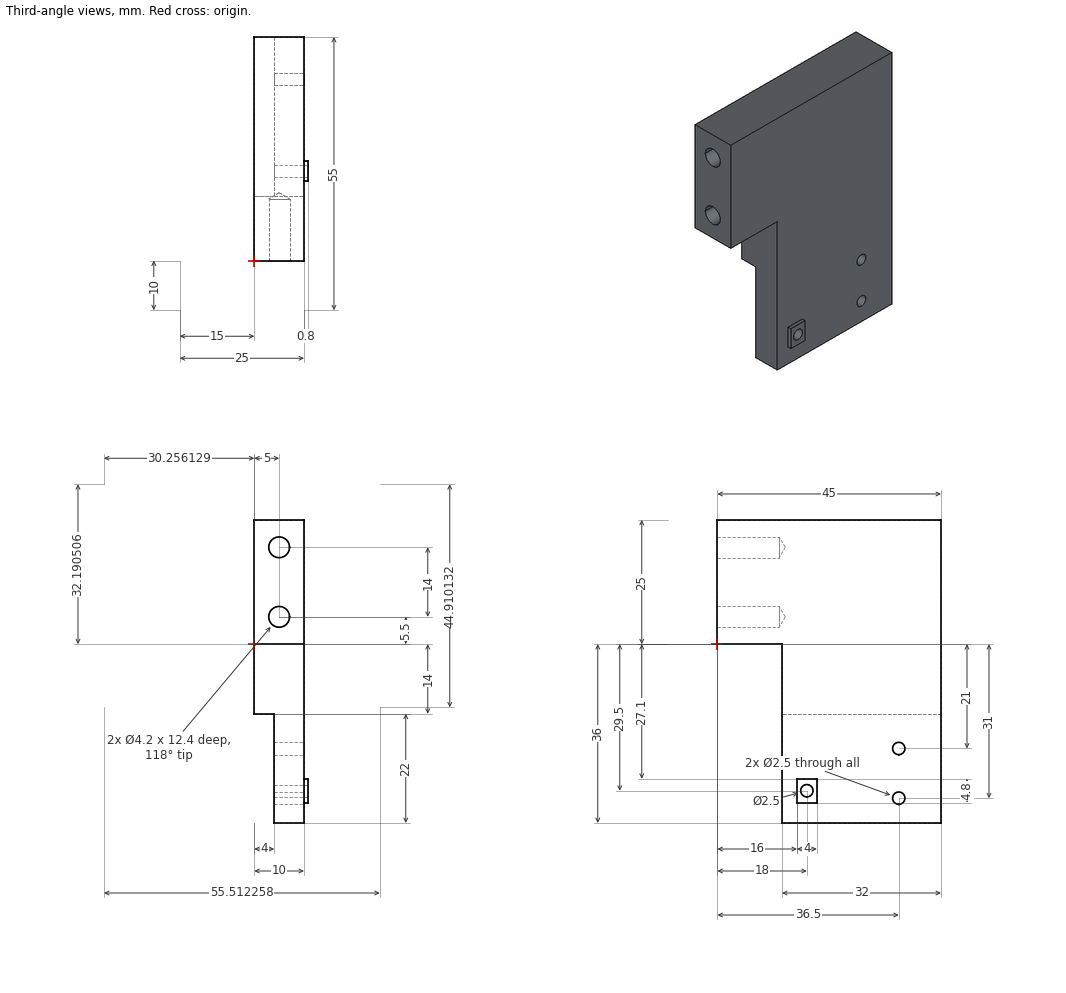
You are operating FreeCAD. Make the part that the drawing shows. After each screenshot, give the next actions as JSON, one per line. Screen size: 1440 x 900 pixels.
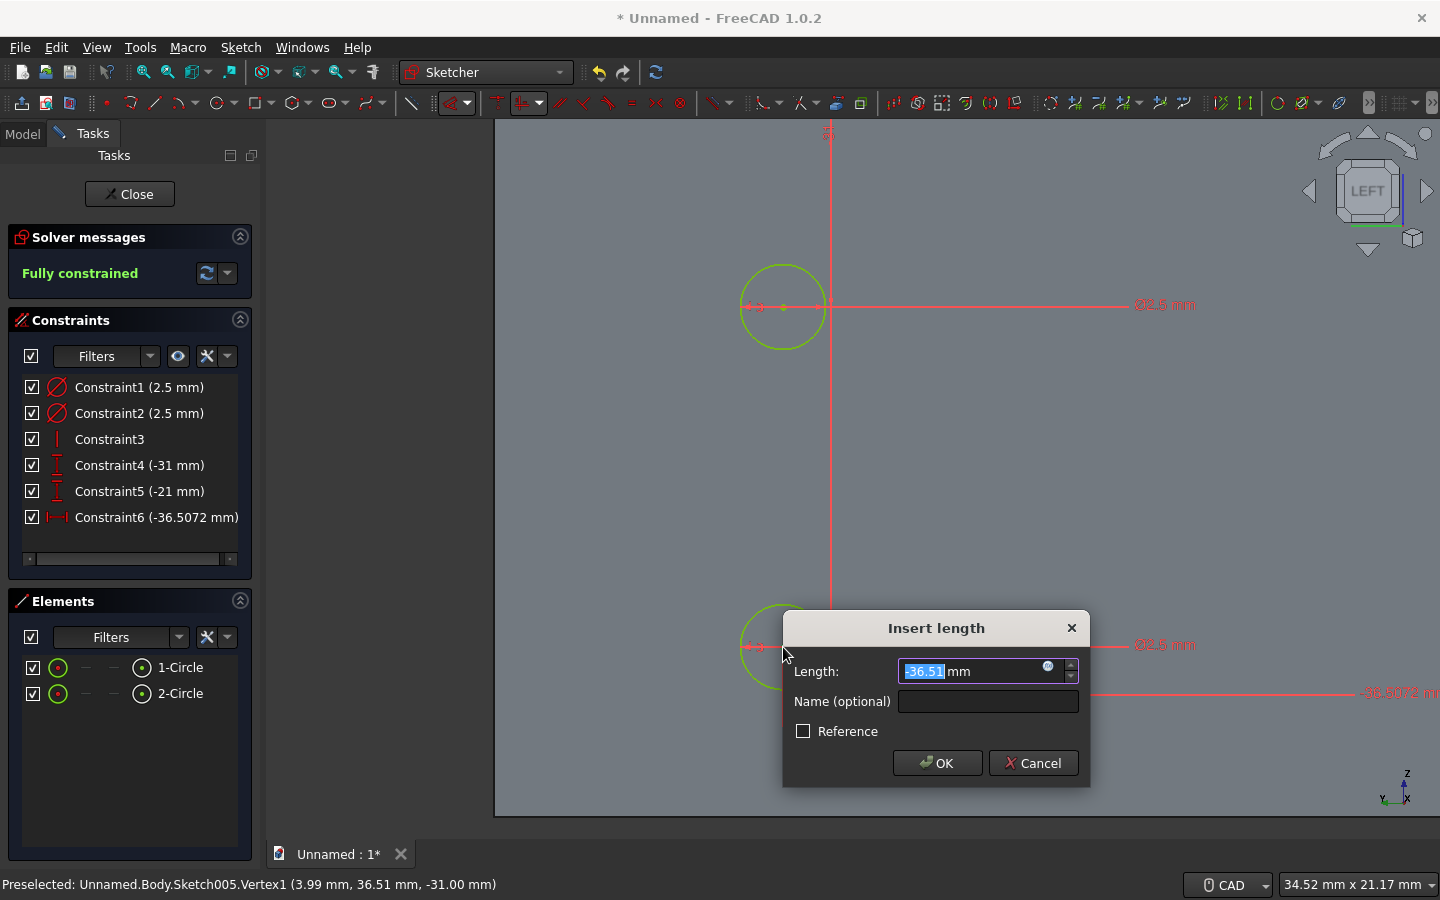
{"action": "type", "text": "-36.5"}
{"action": "key", "text": "Return"}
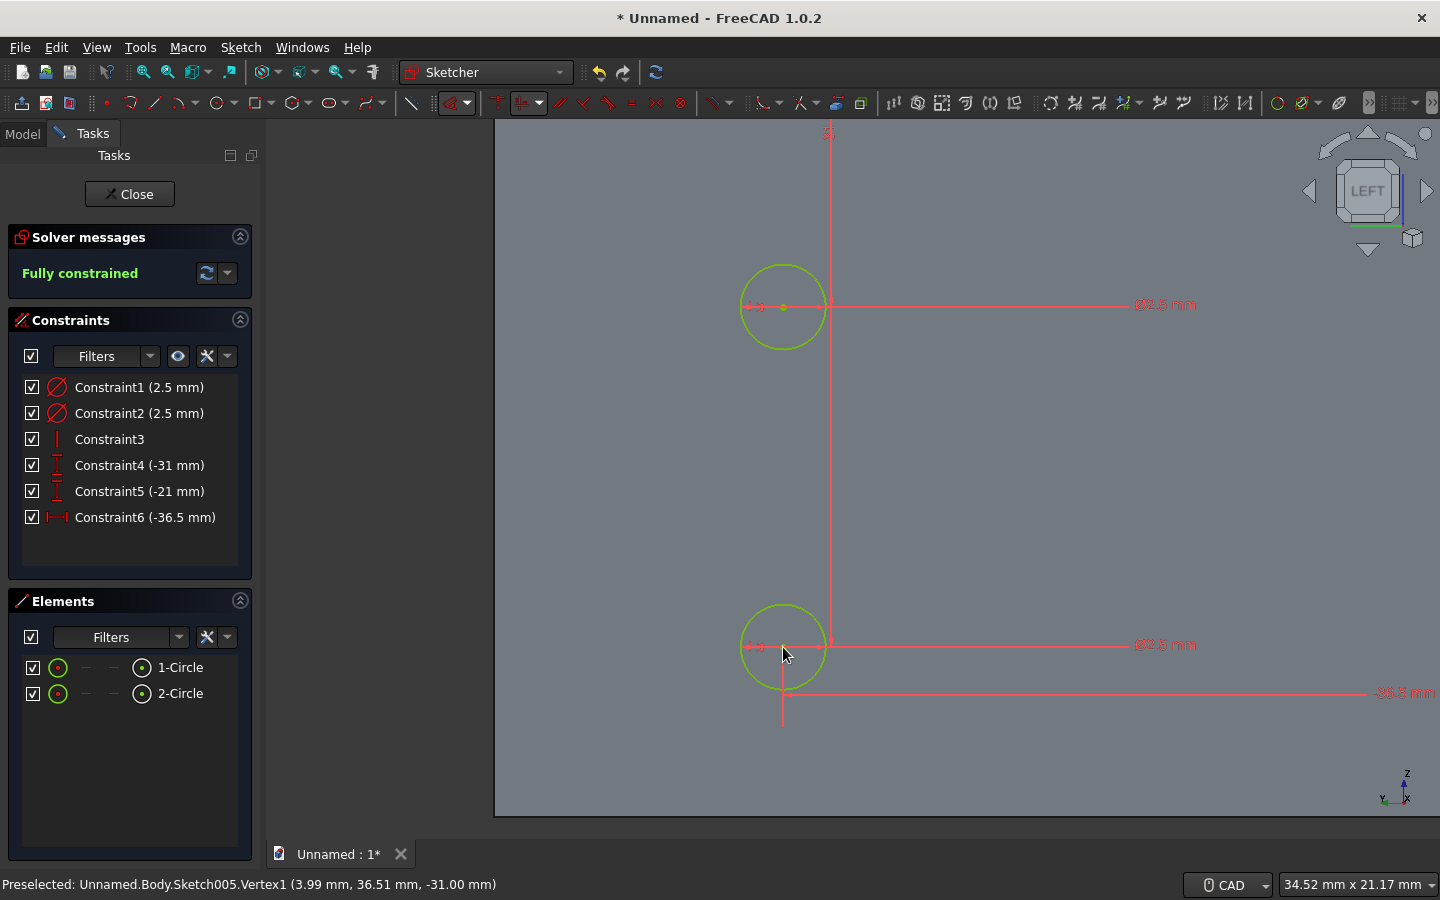
{"action": "left_click", "coordinate": [130, 194]}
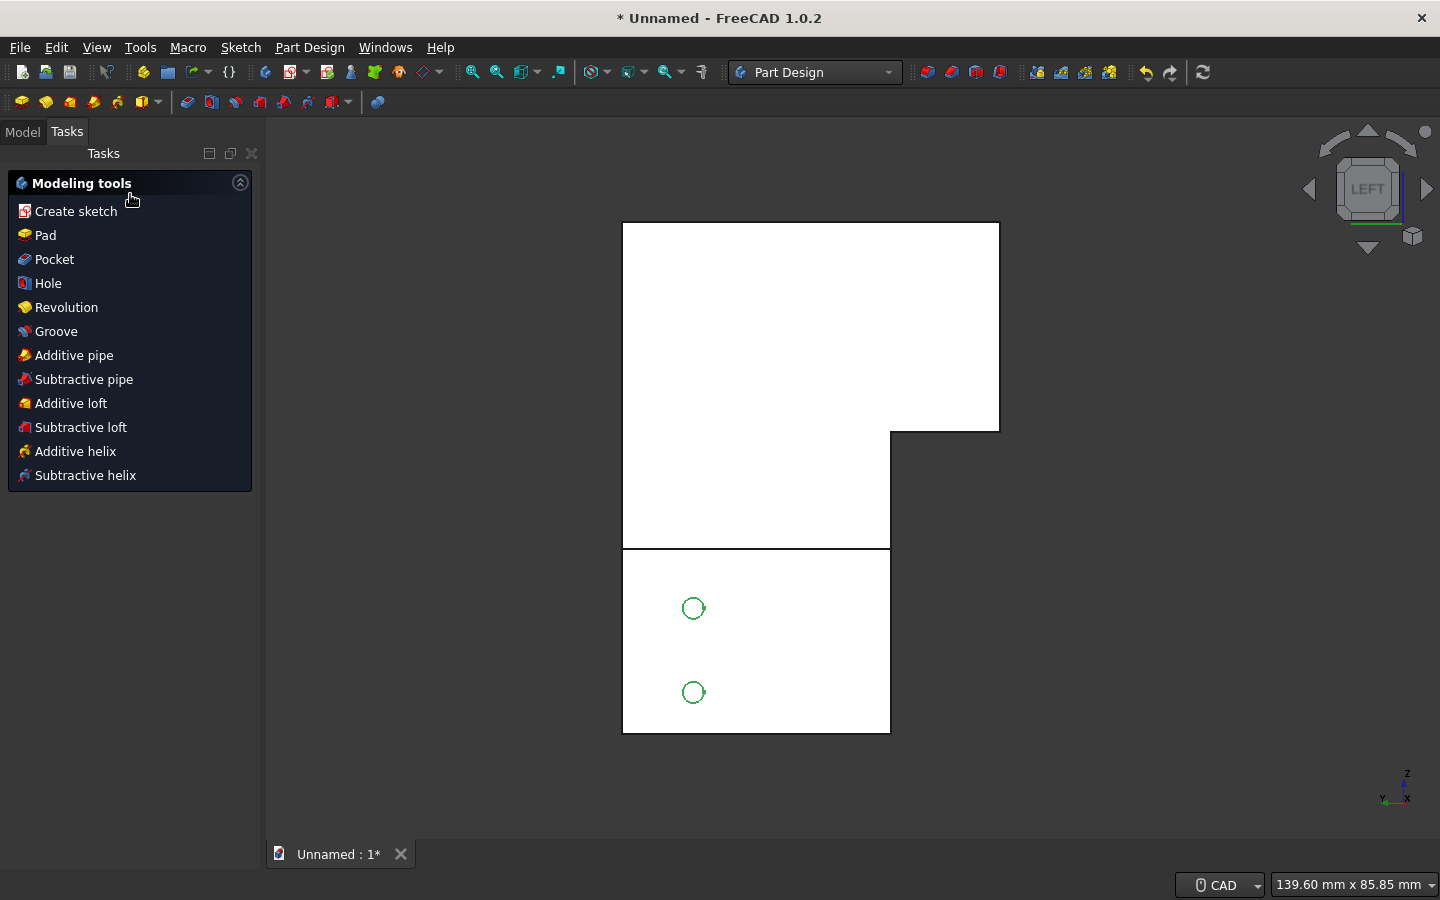
{"action": "left_click", "coordinate": [212, 102]}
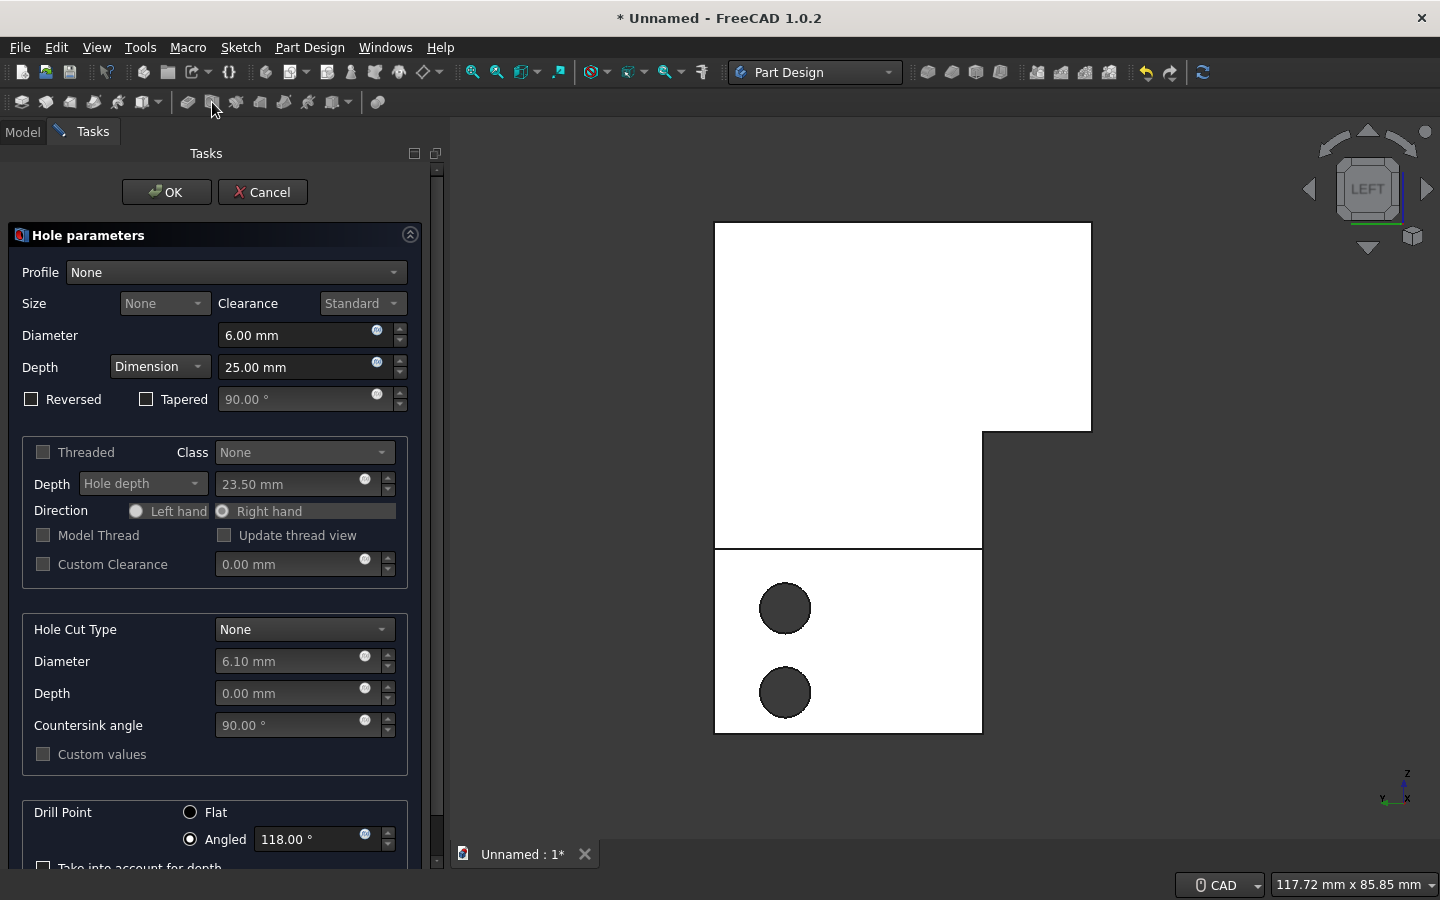
{"action": "triple_click", "coordinate": [305, 335]}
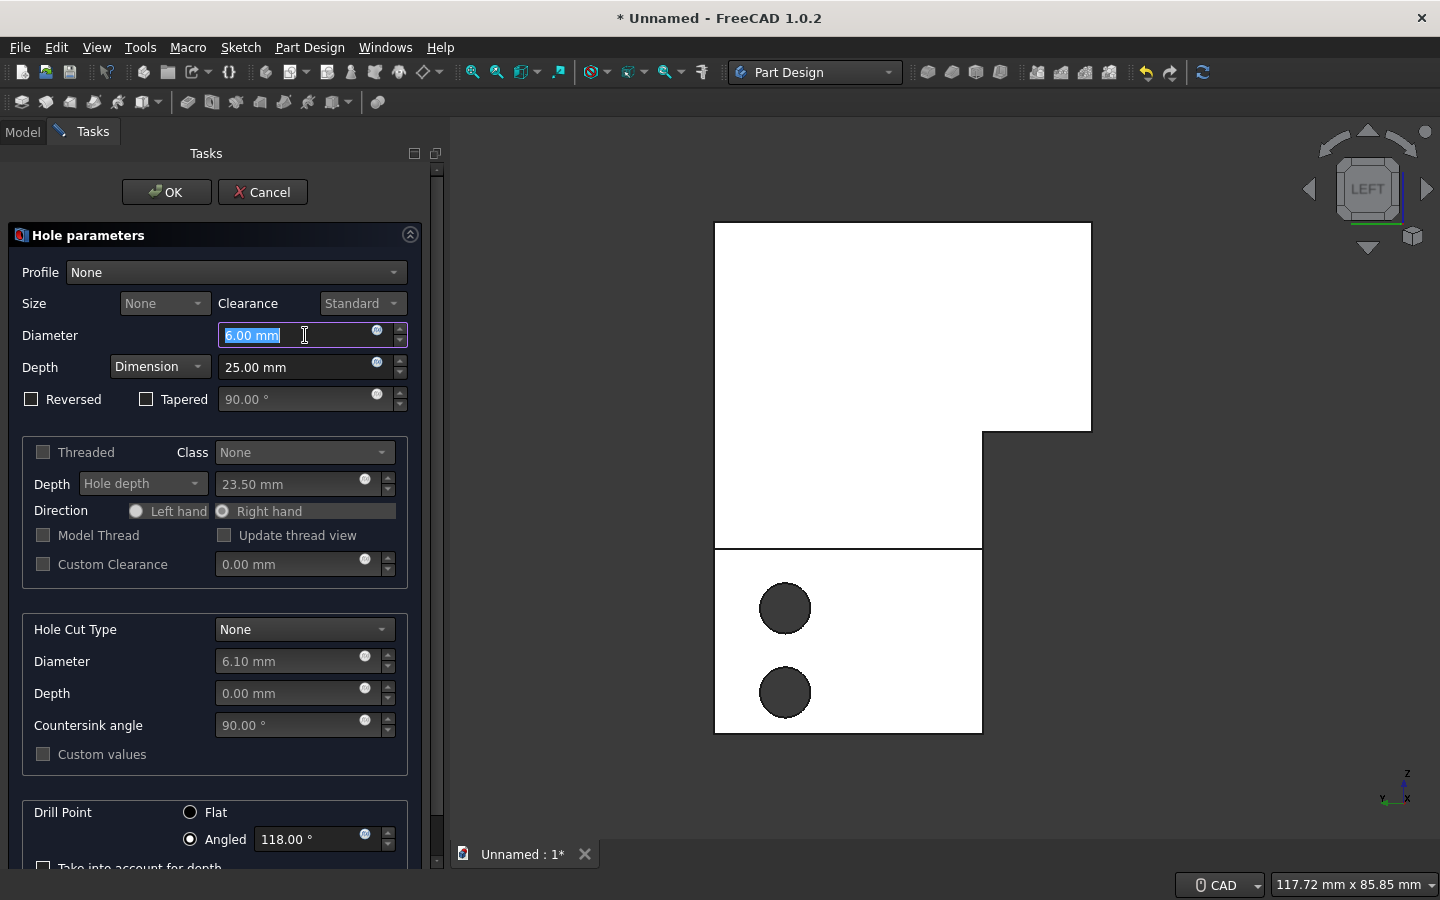
{"action": "type", "text": "2.5"}
{"action": "key", "text": "Tab"}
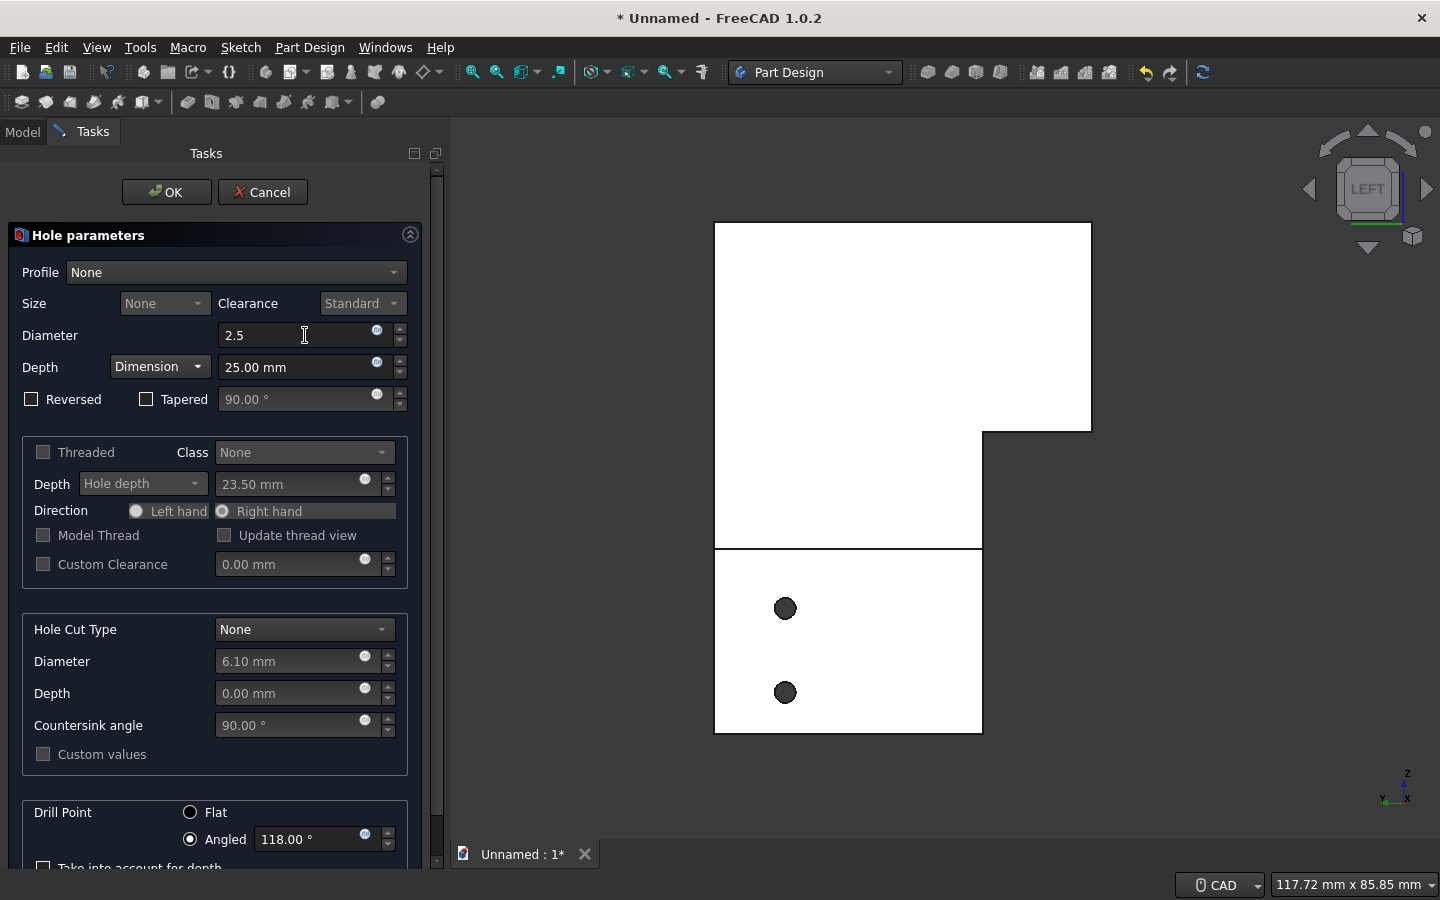
{"action": "left_click", "coordinate": [161, 366]}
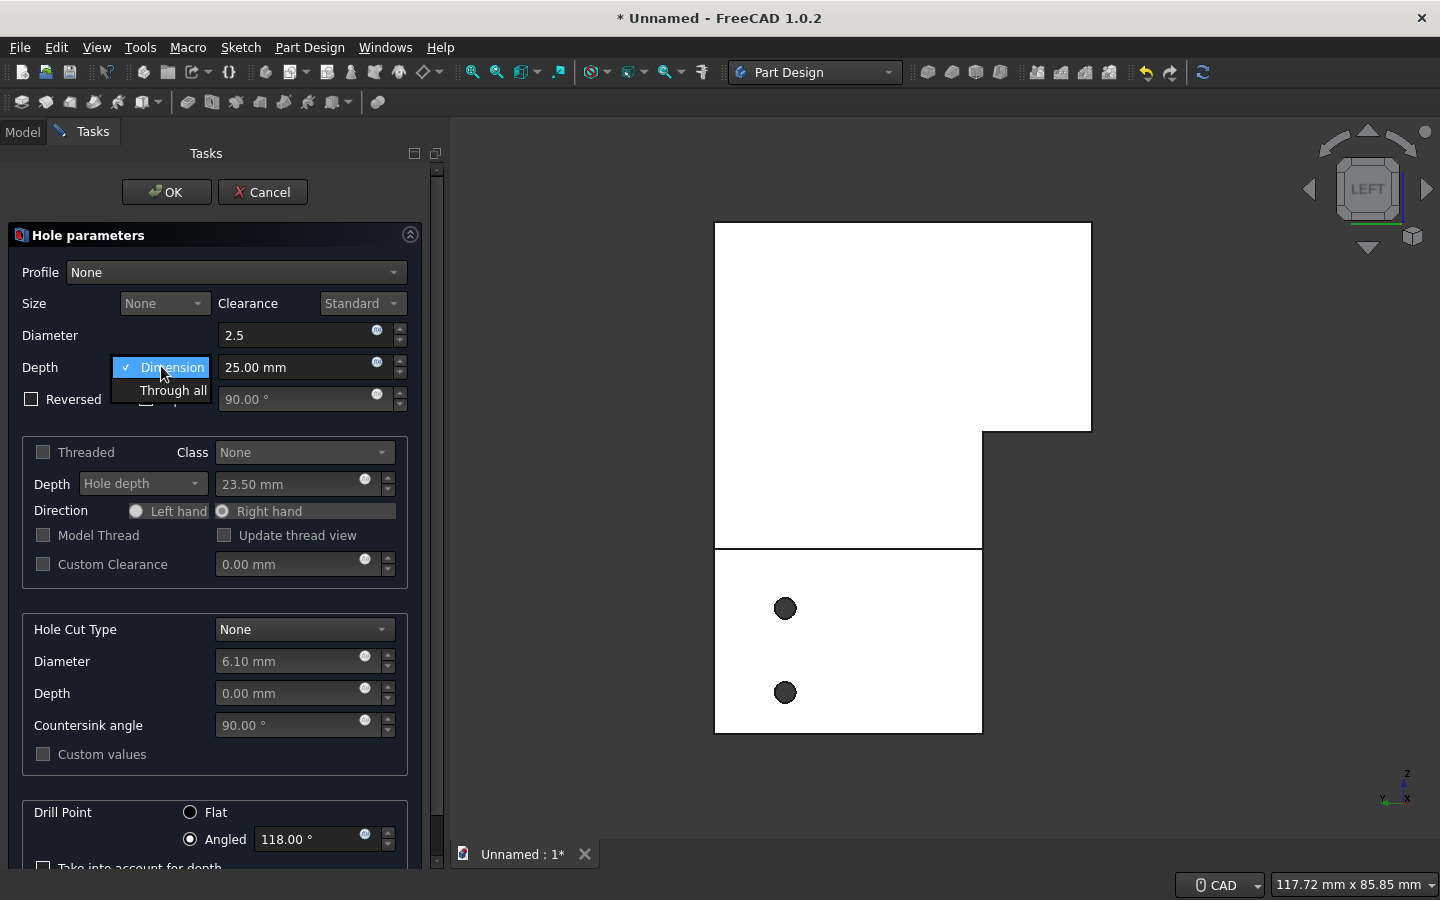
{"action": "left_click", "coordinate": [160, 390]}